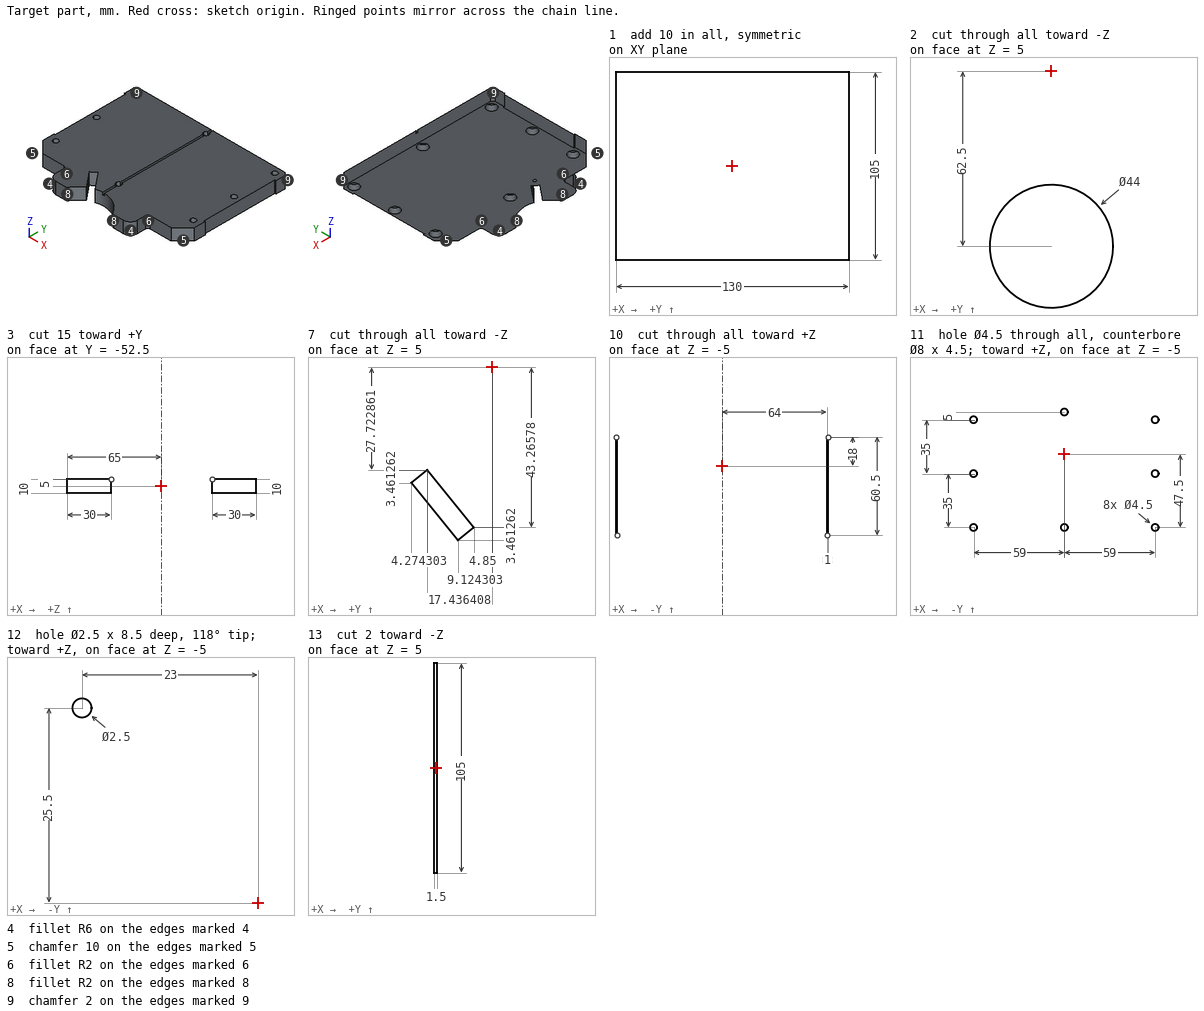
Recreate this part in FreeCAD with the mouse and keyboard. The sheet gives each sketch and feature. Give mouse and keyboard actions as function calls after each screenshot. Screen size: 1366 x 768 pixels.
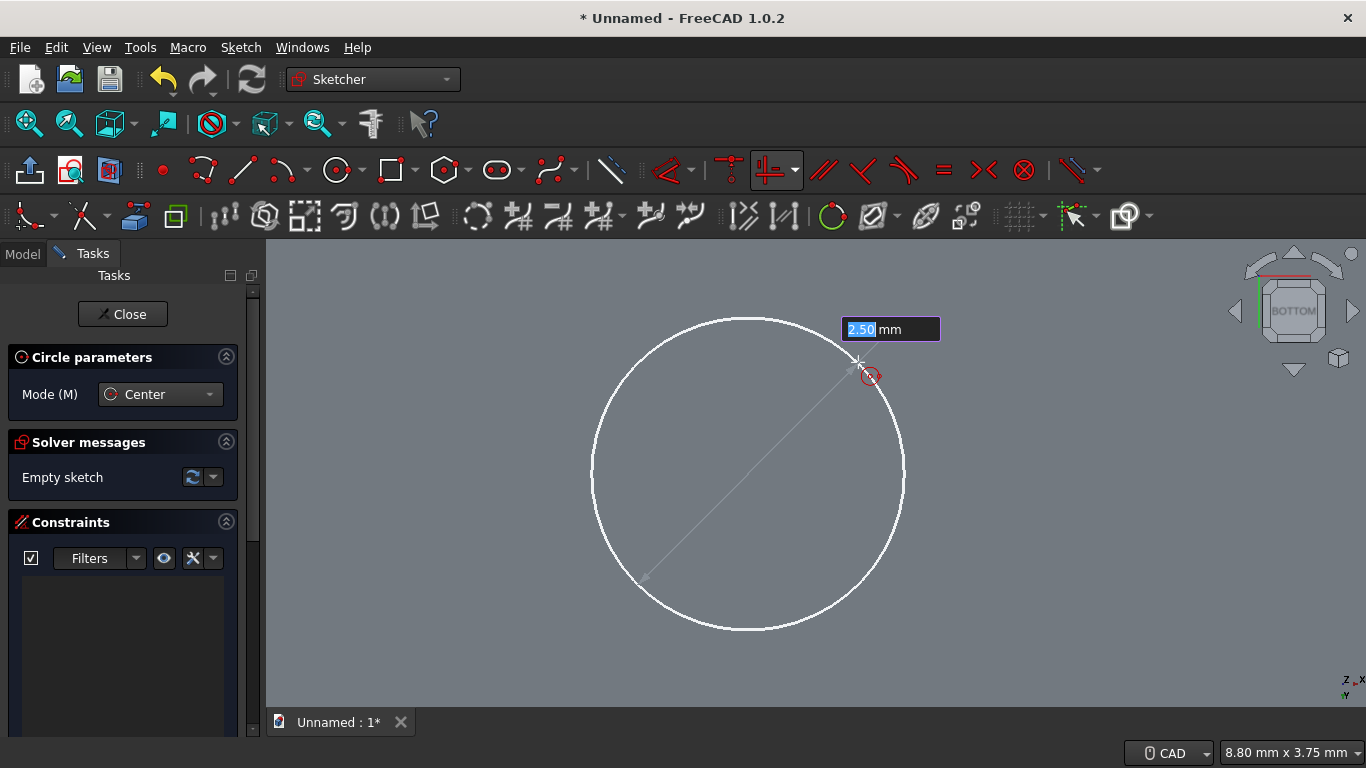
text(2.5)
key(Return)
key(Escape)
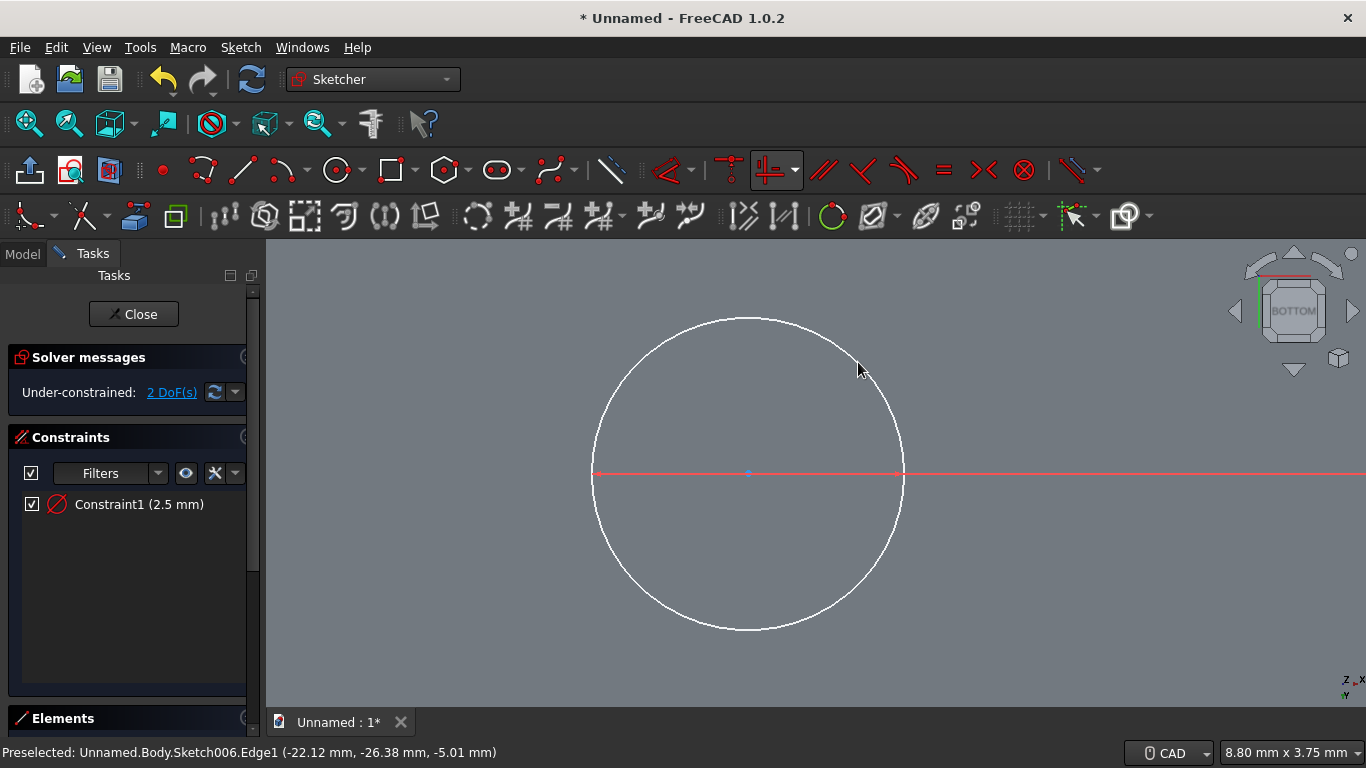
click(666, 170)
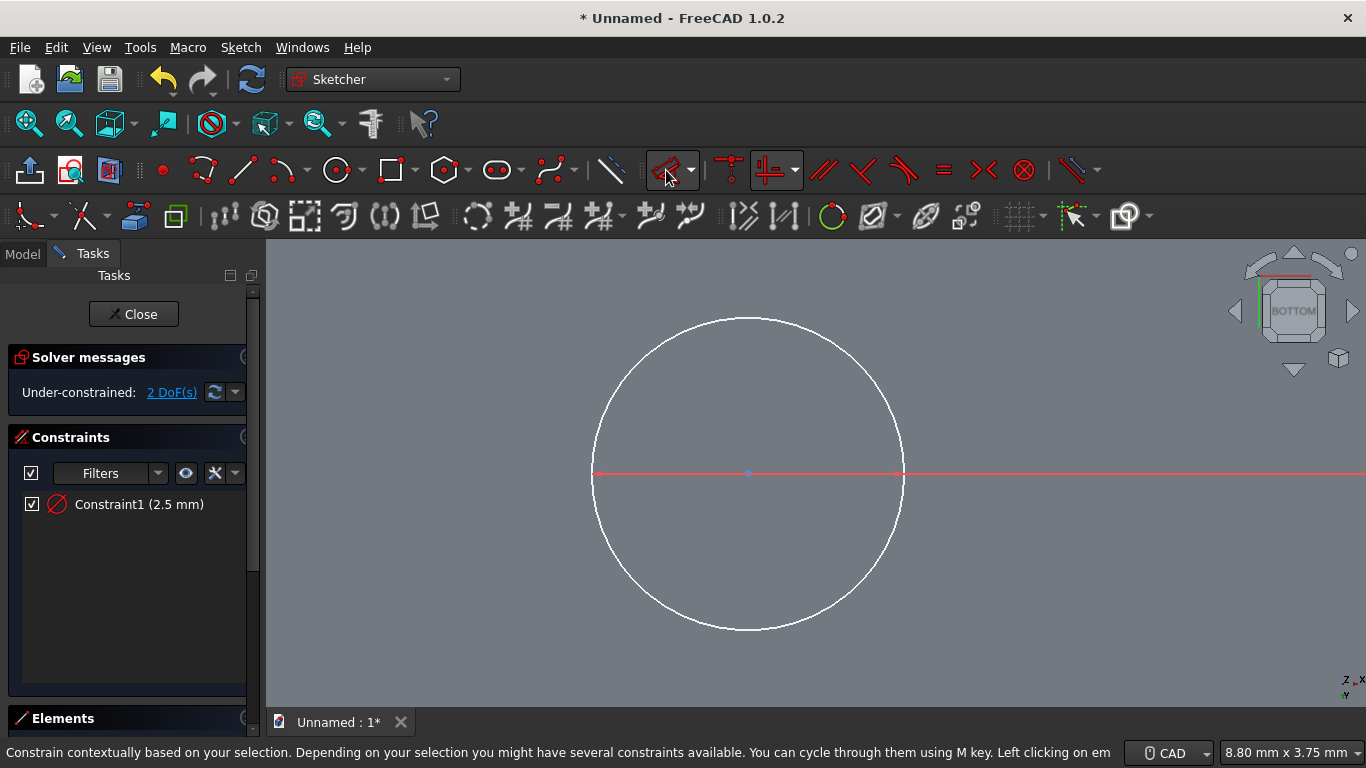
click(748, 474)
click(975, 440)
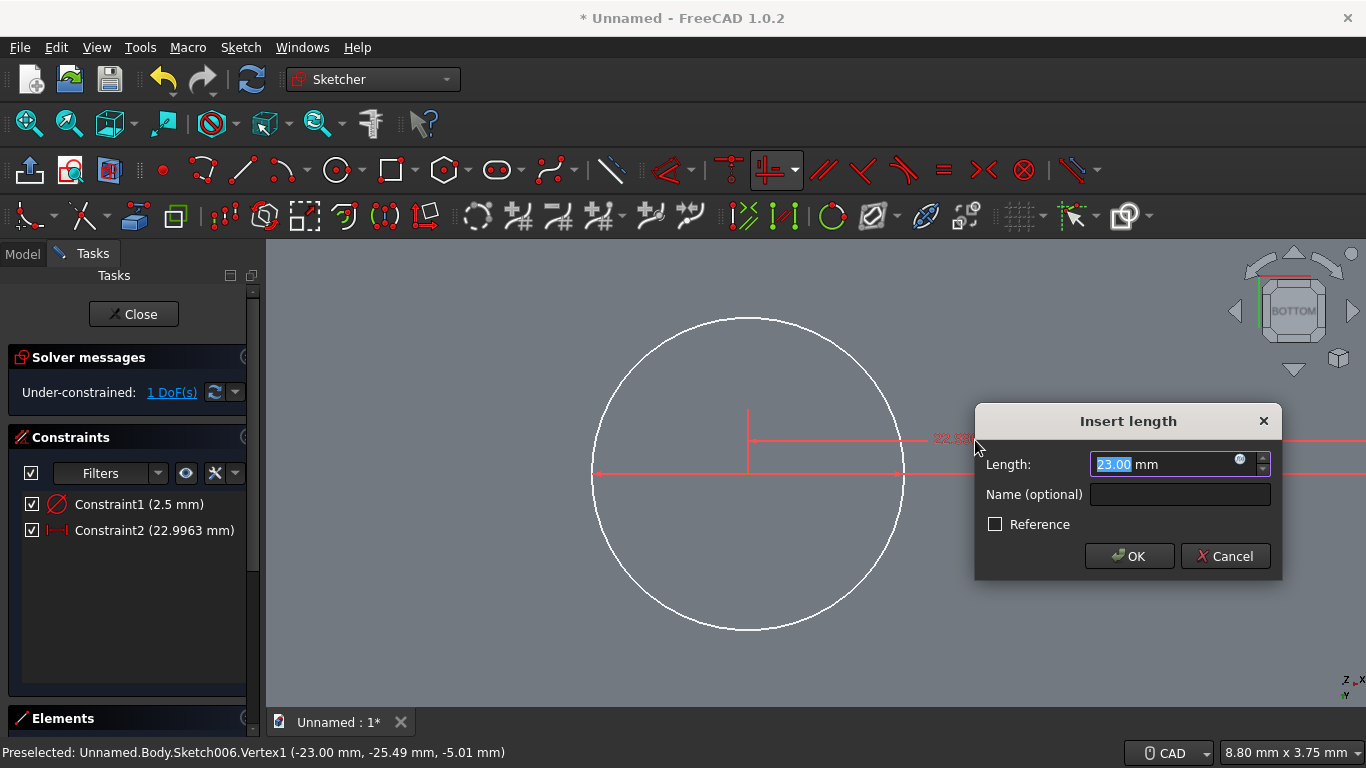
text(23)
key(Return)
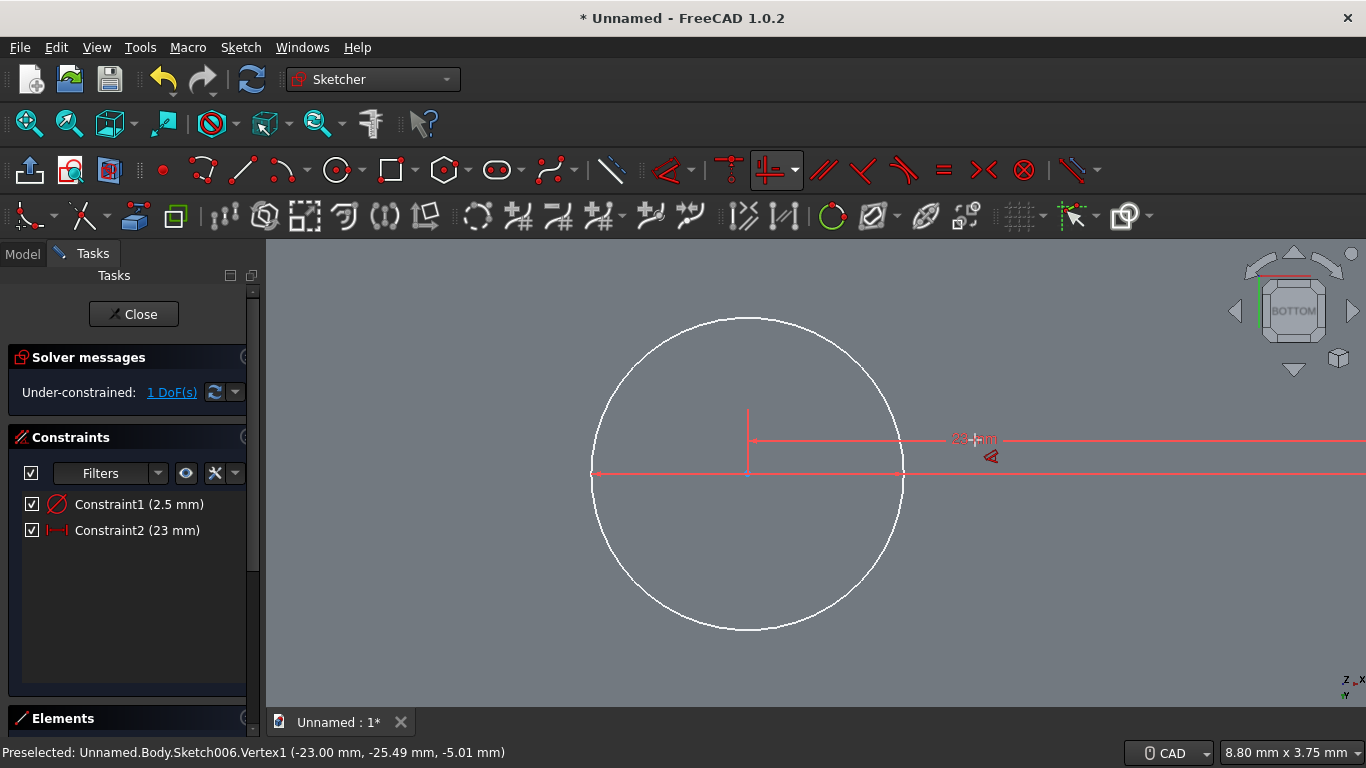
click(748, 474)
click(714, 576)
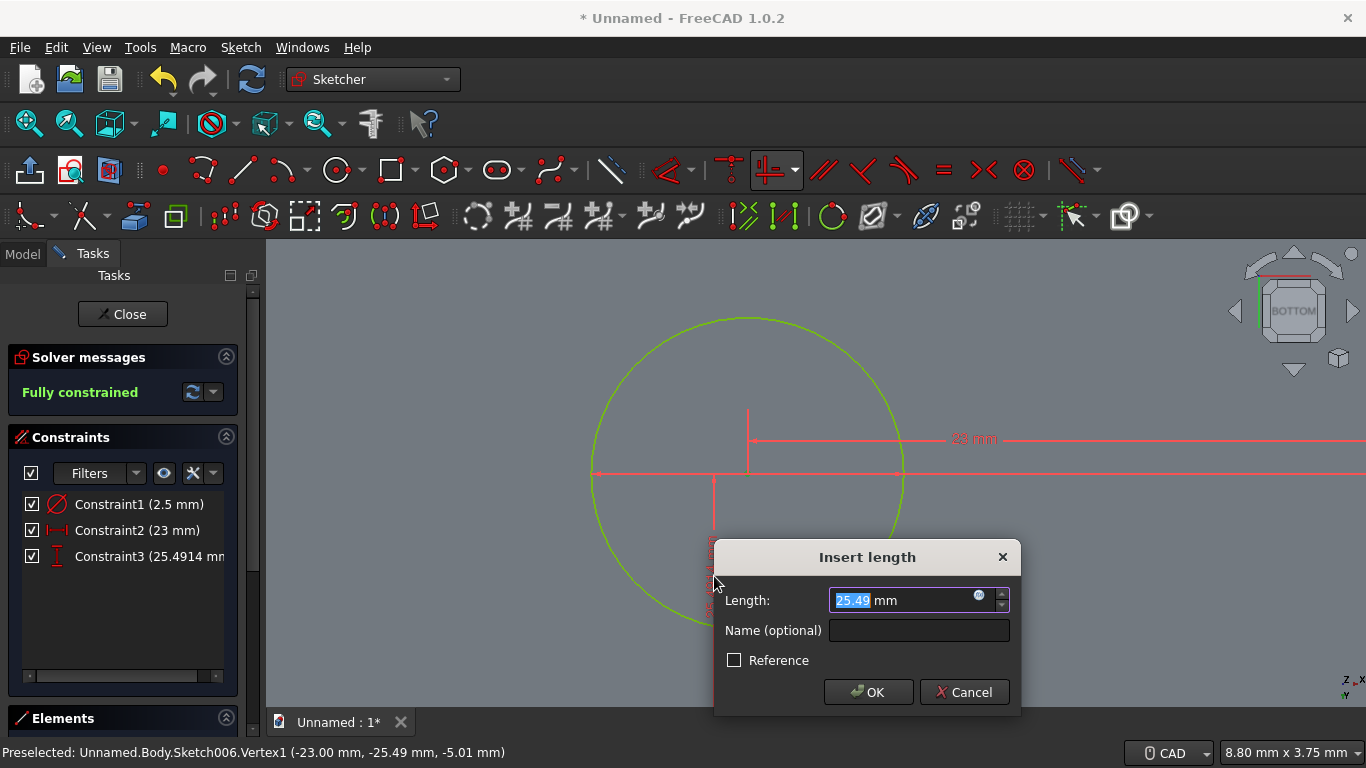
text(25.5)
key(Return)
key(Escape)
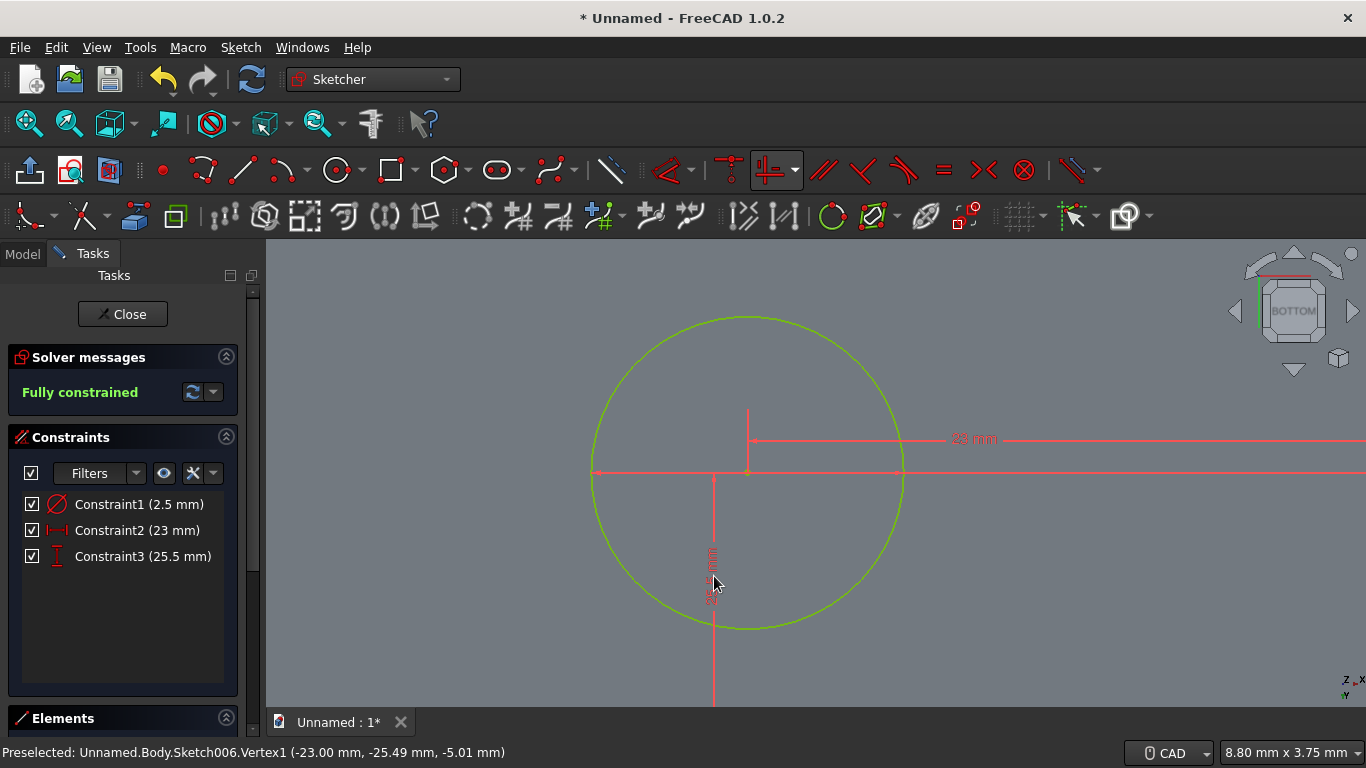
click(123, 314)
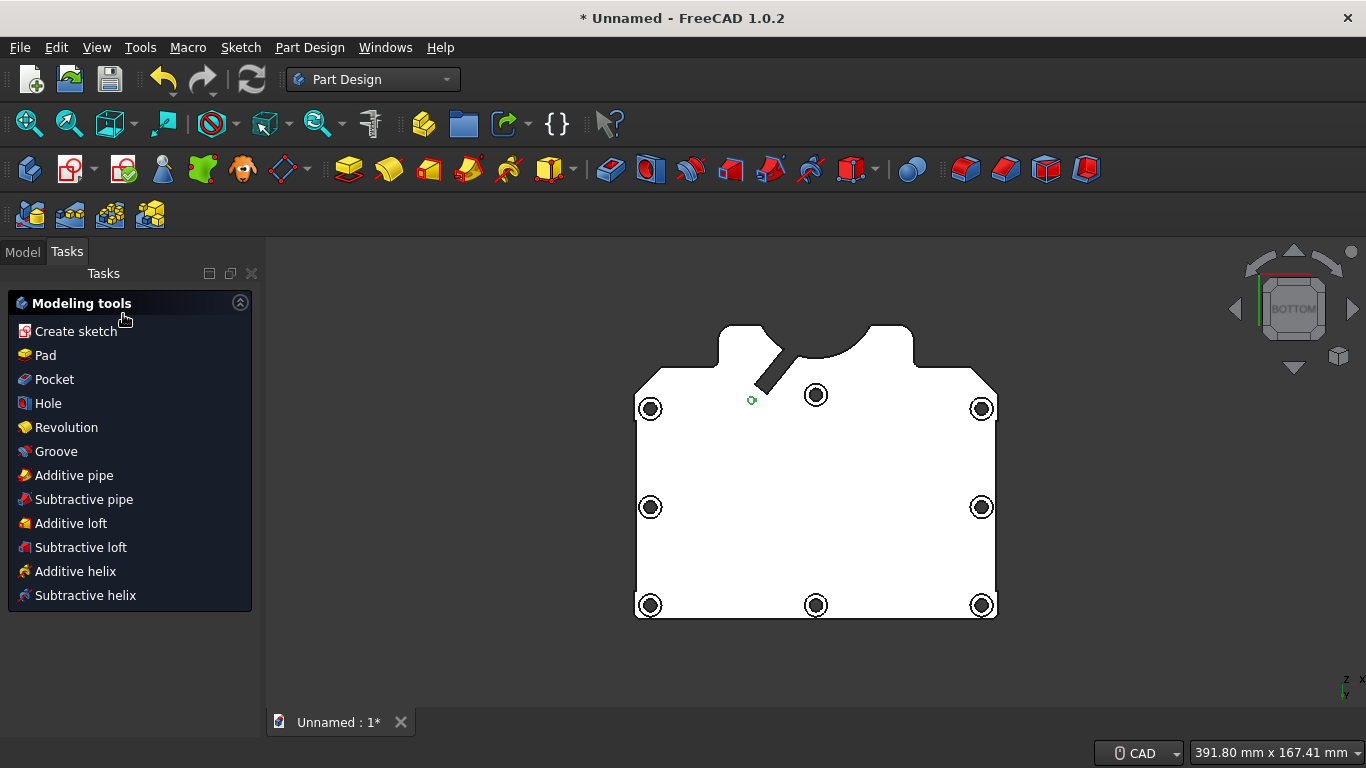
click(652, 170)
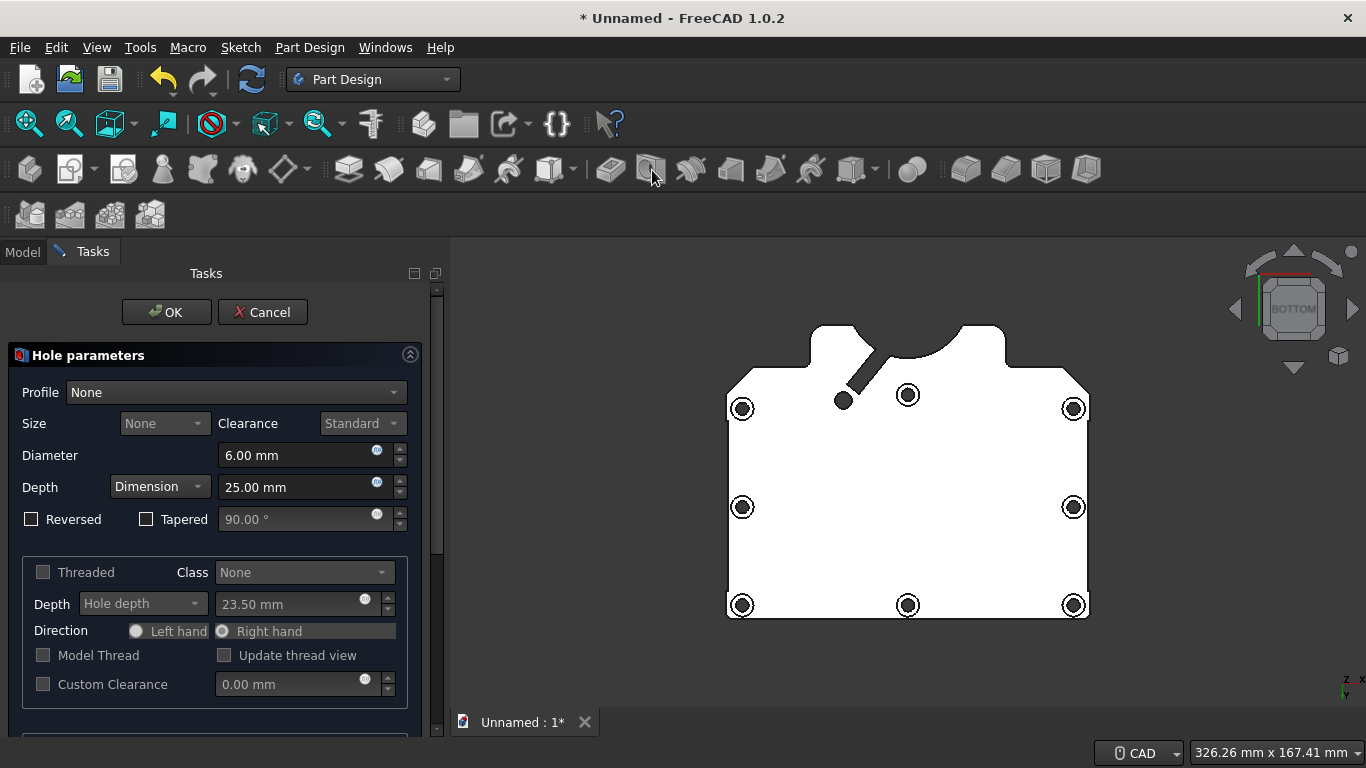
triple_click(305, 455)